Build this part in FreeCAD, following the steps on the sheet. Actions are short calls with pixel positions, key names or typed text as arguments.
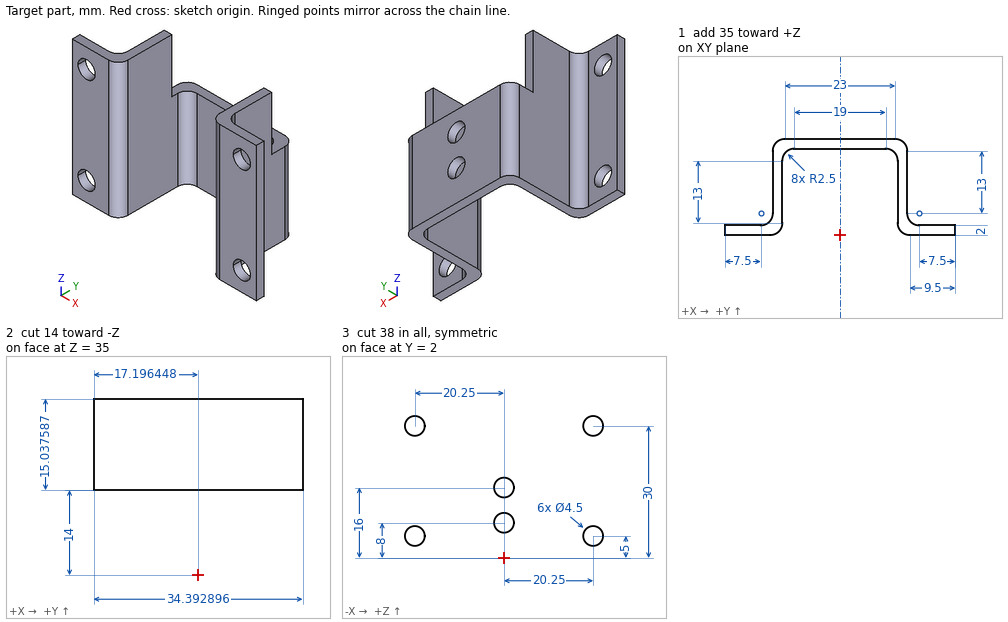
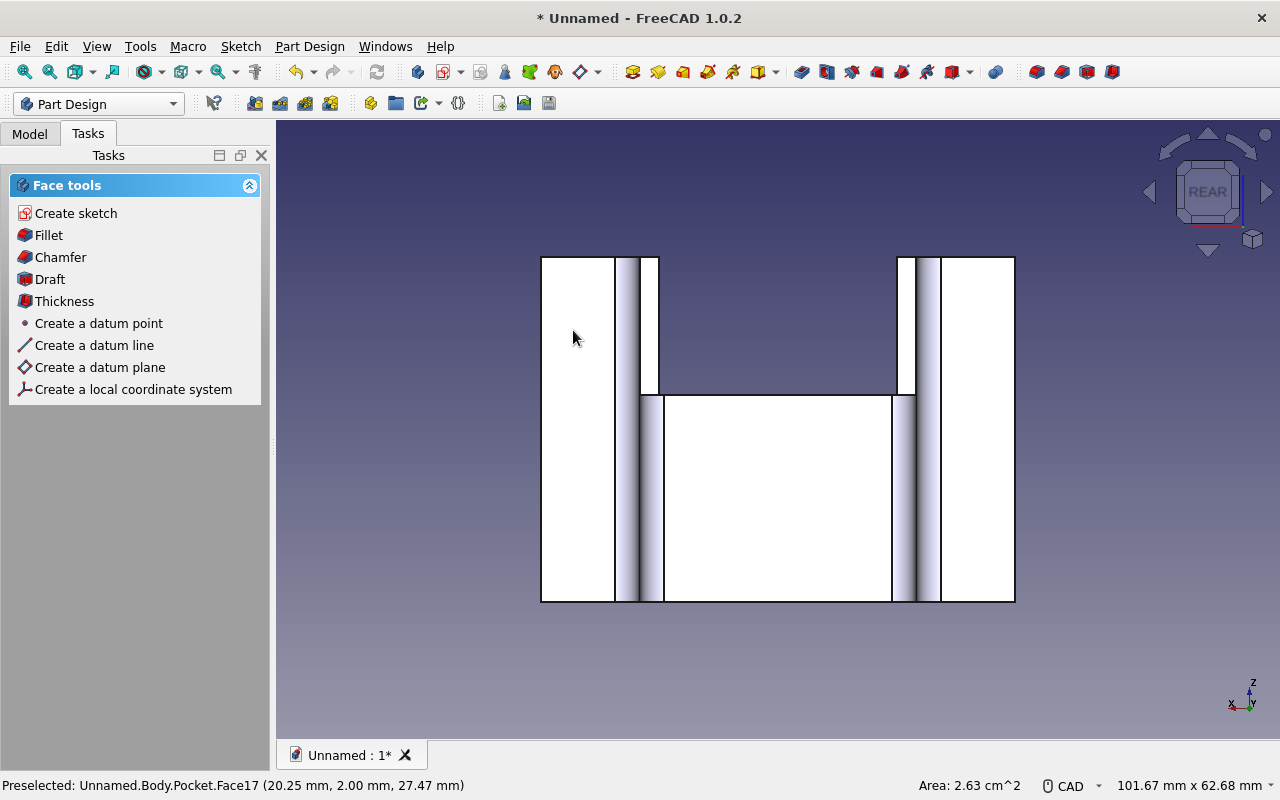
click(442, 72)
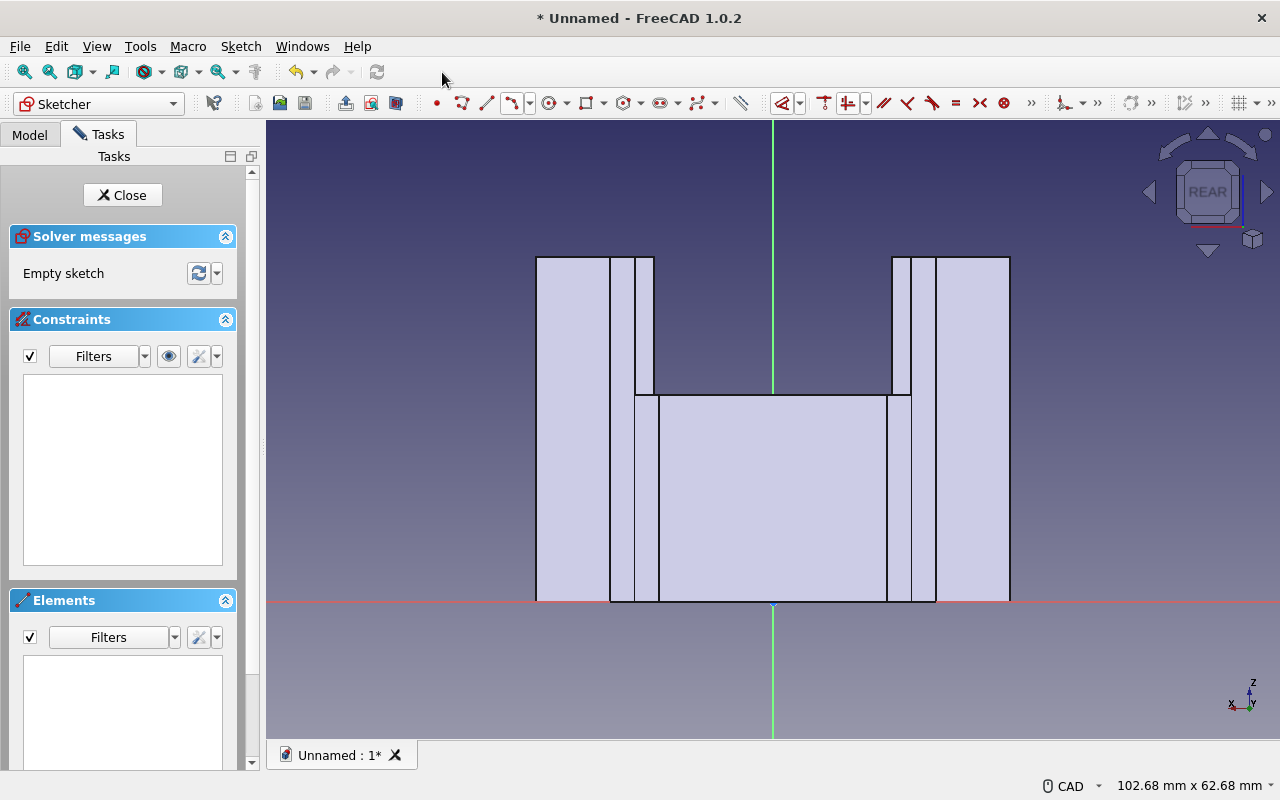
click(396, 104)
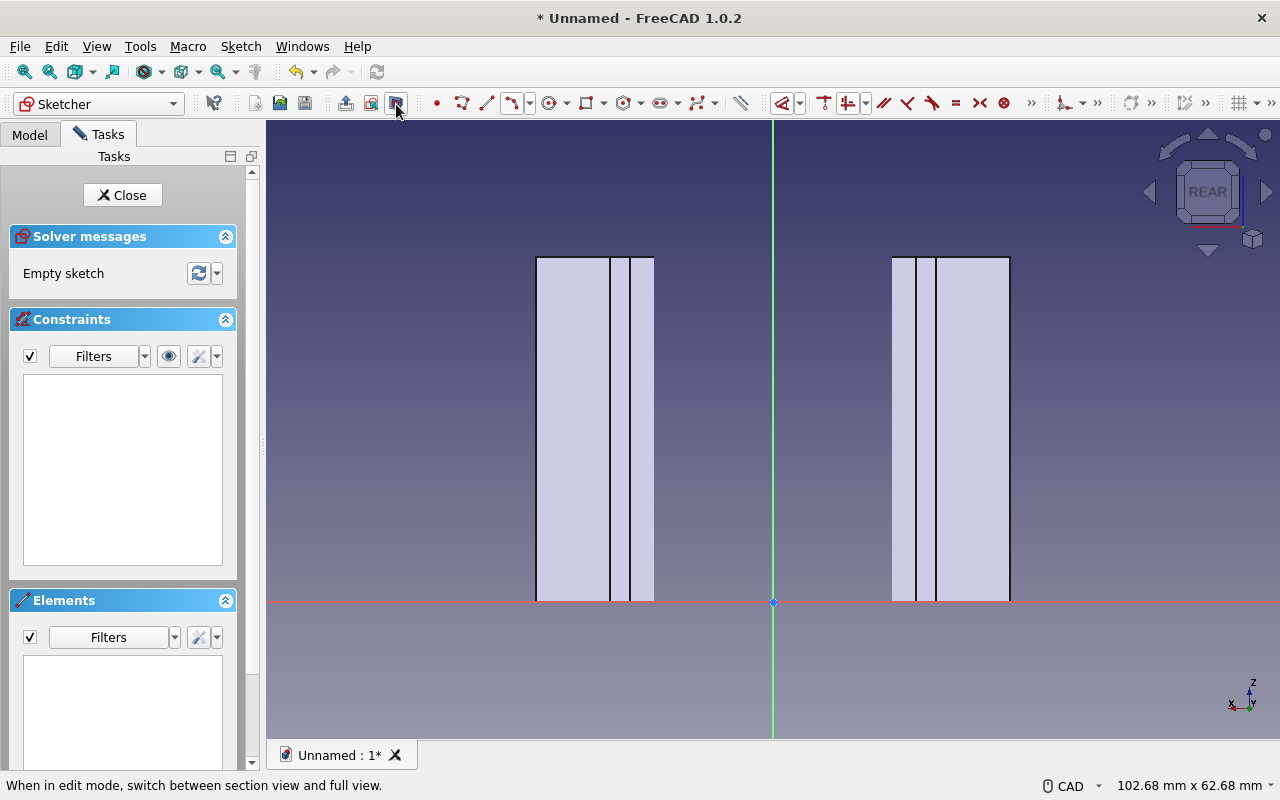
click(548, 104)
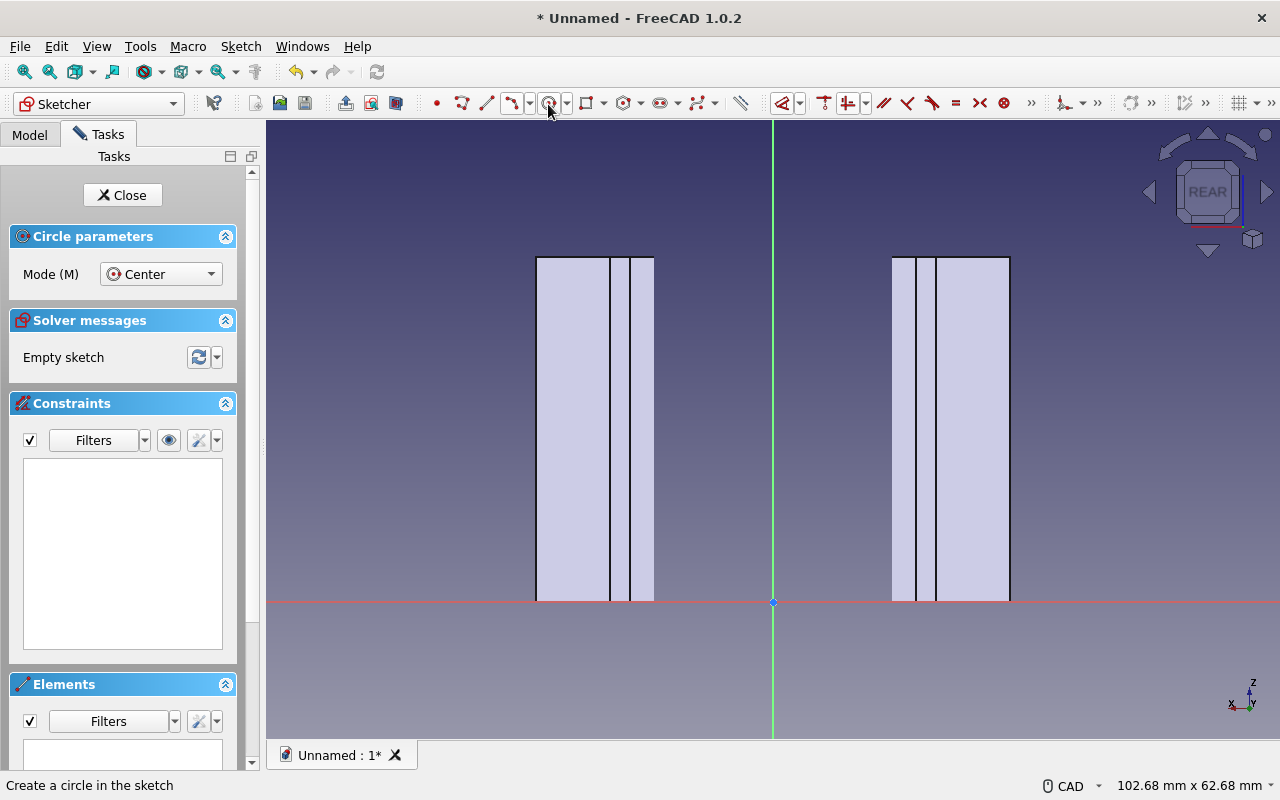
click(973, 553)
click(989, 537)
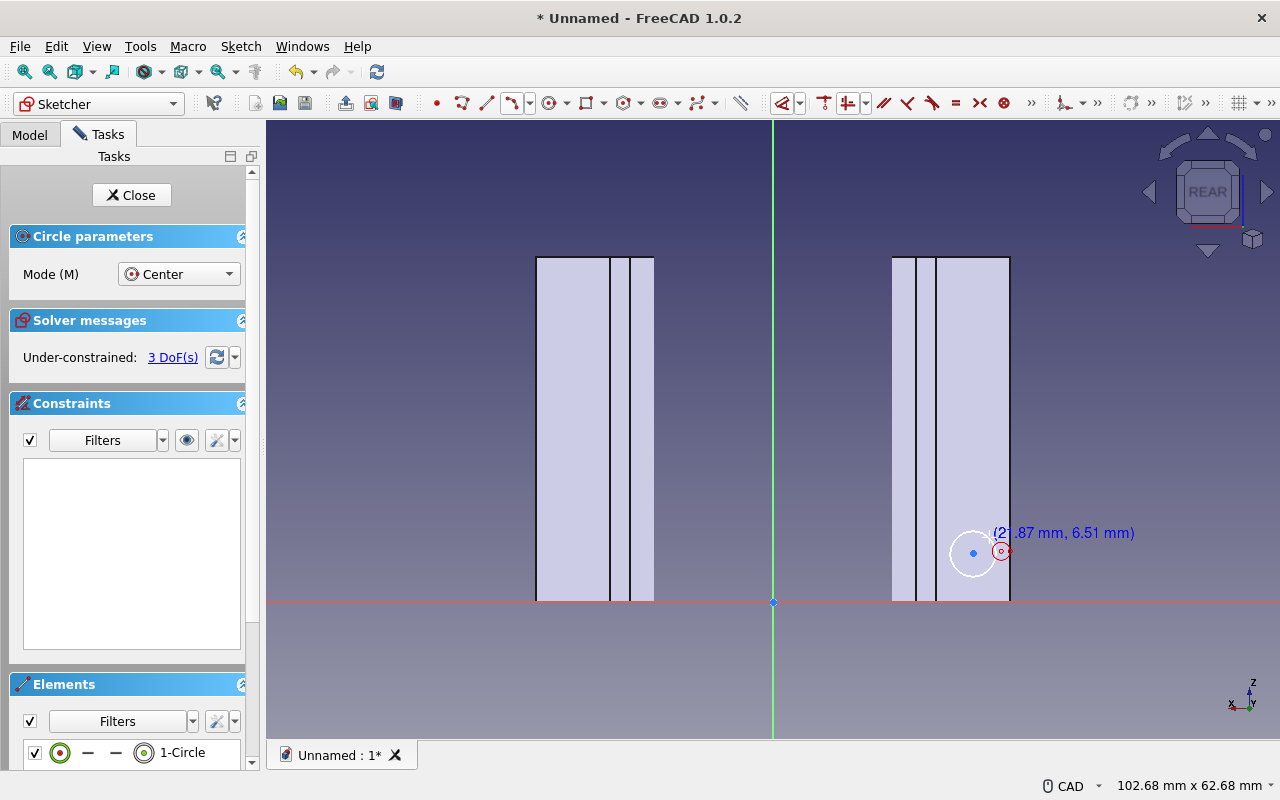
click(973, 306)
click(989, 290)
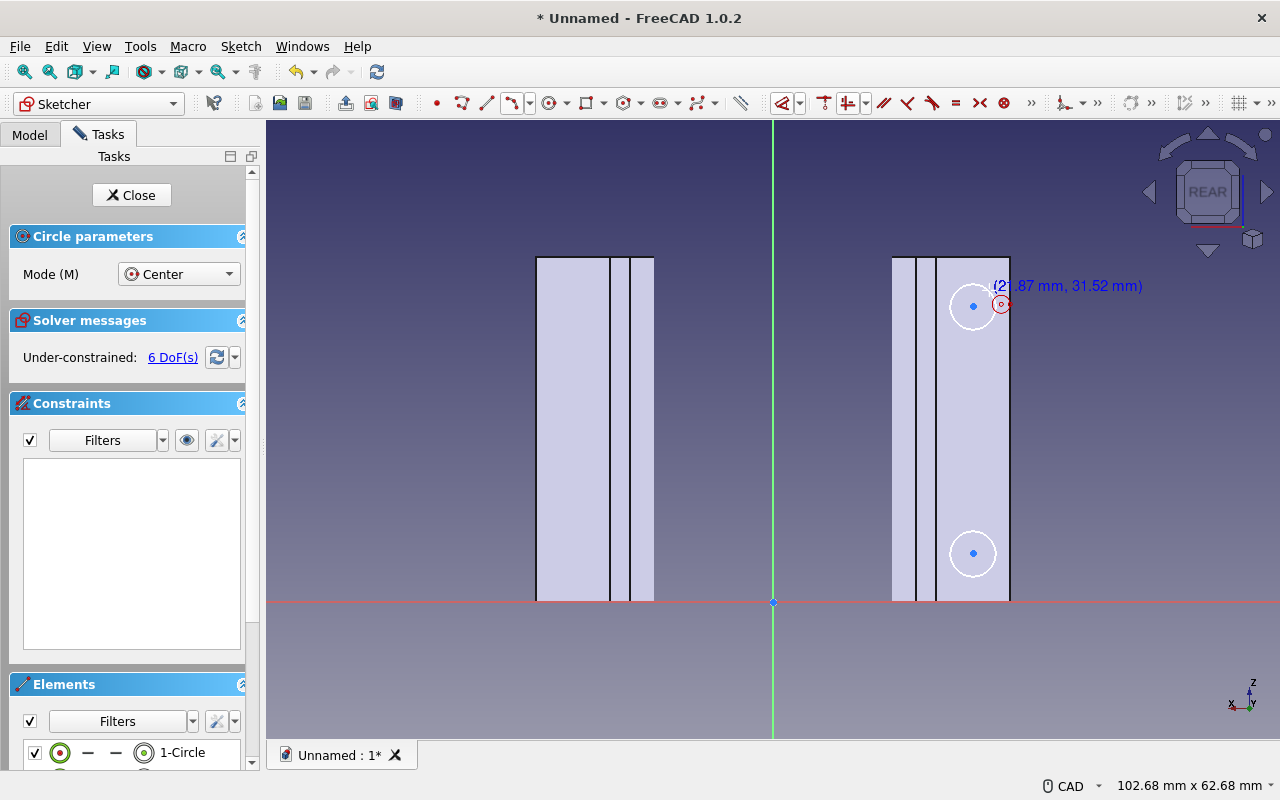
click(573, 306)
click(589, 290)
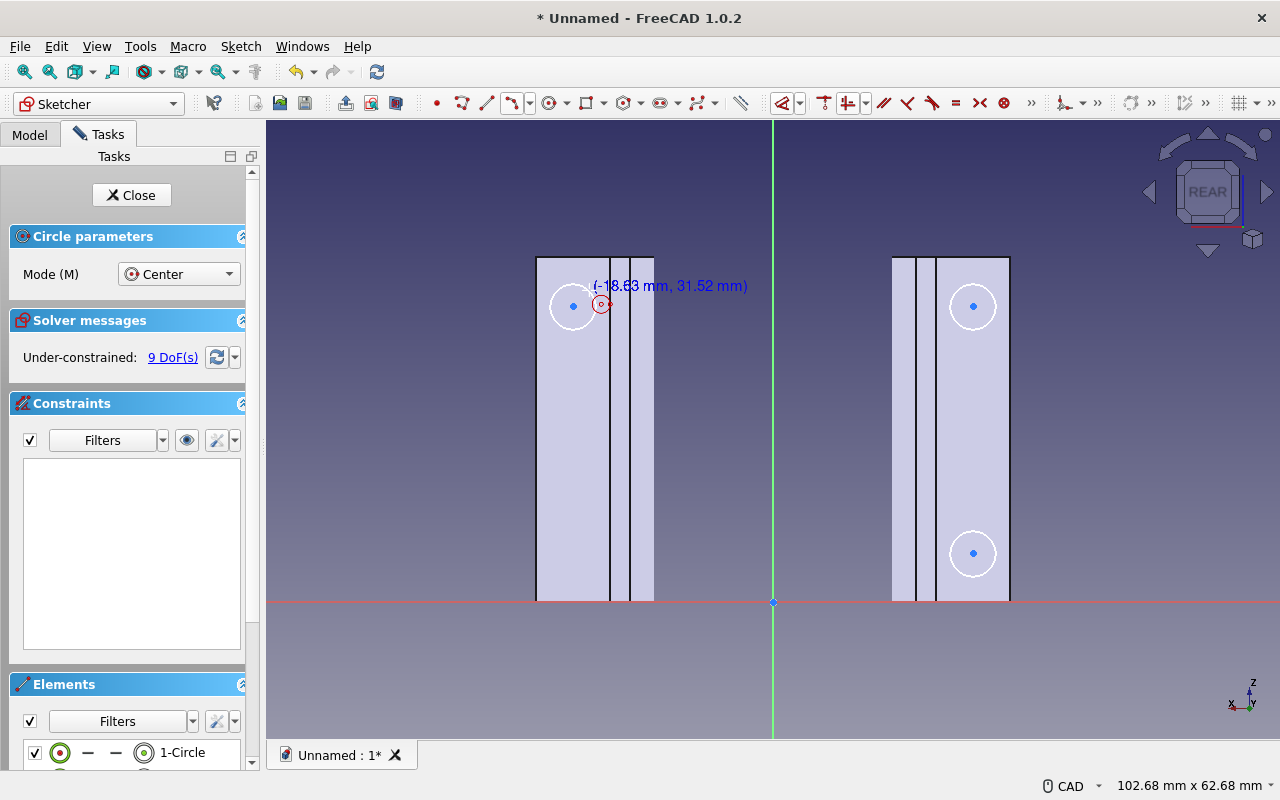
click(573, 553)
click(589, 537)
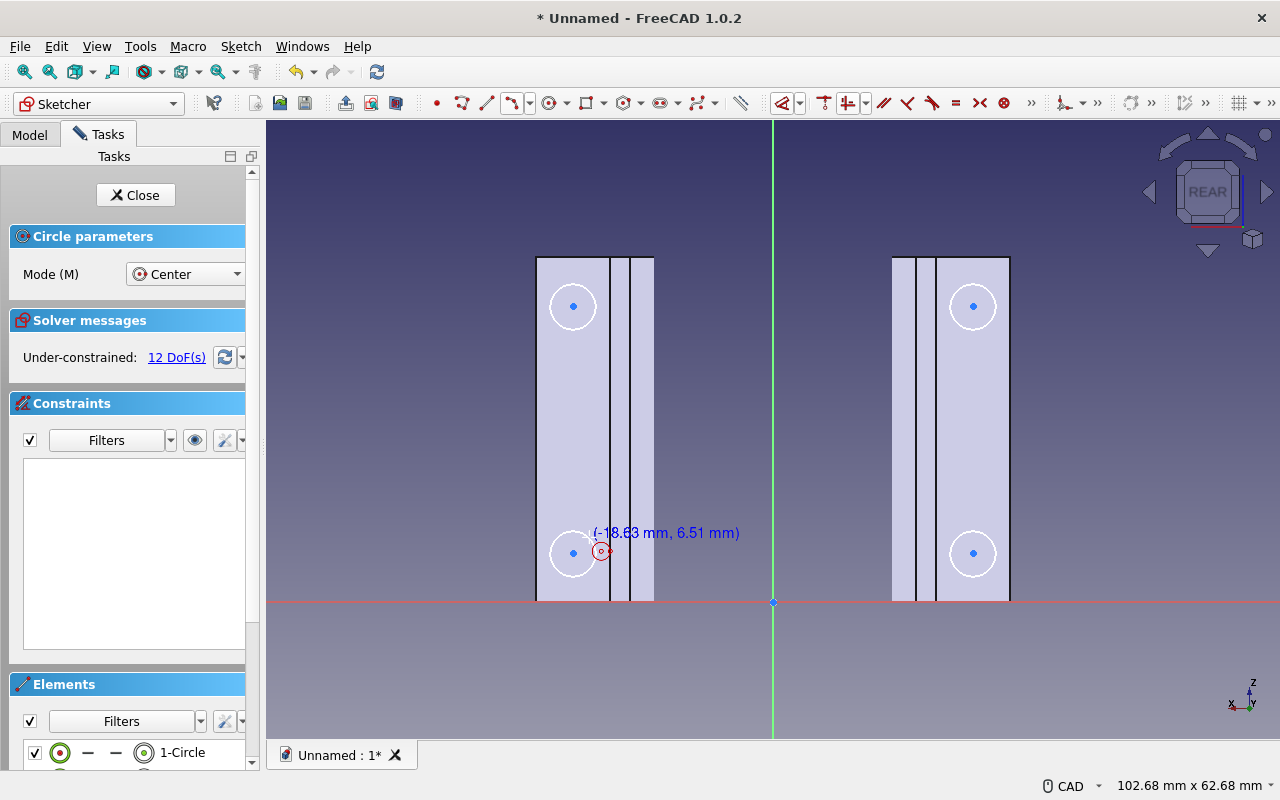
click(773, 523)
click(789, 508)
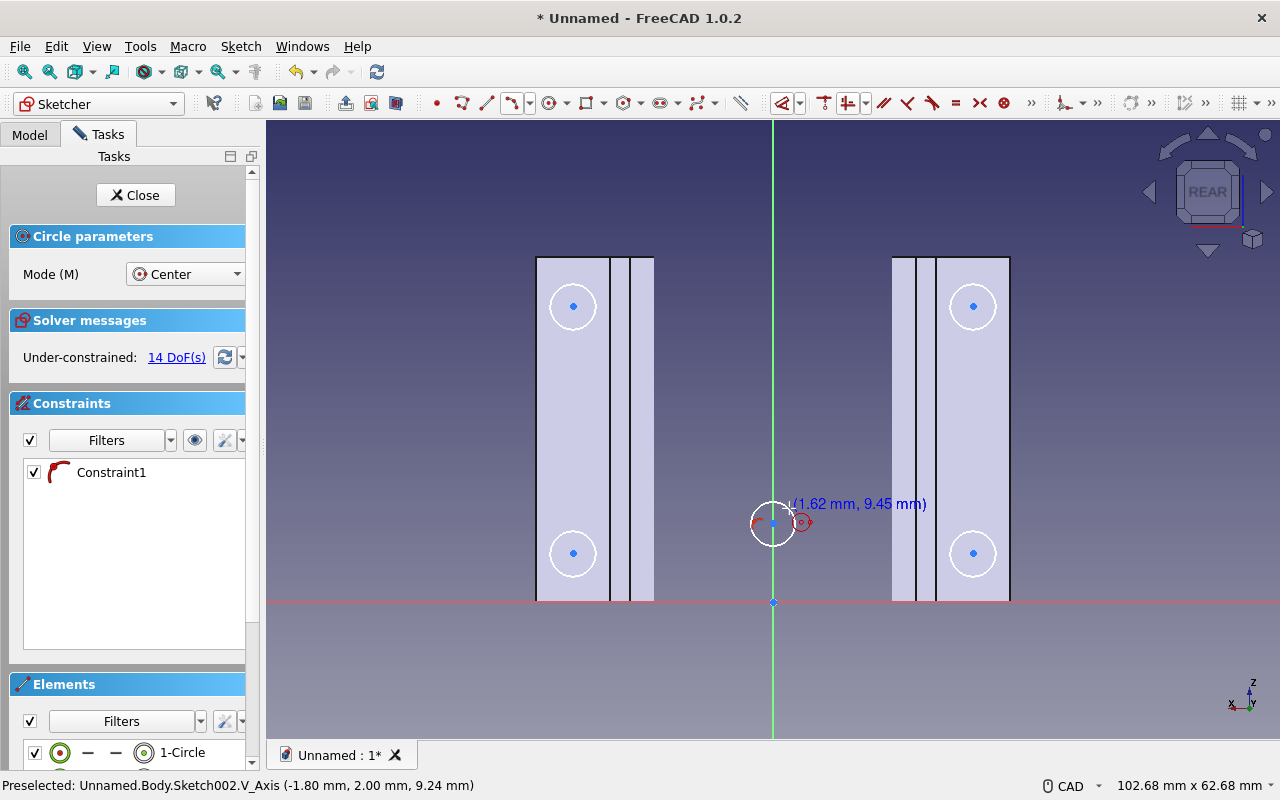
click(773, 444)
click(789, 429)
key(Escape)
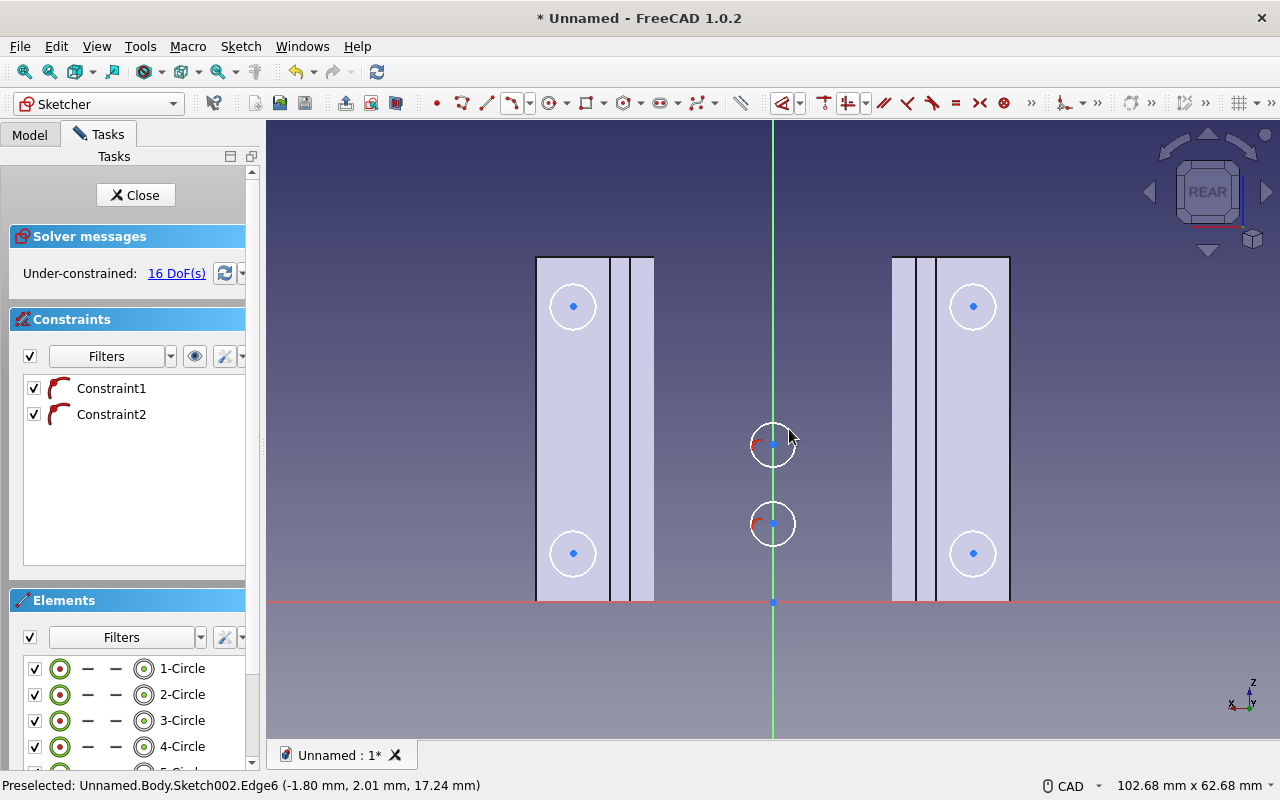
click(989, 538)